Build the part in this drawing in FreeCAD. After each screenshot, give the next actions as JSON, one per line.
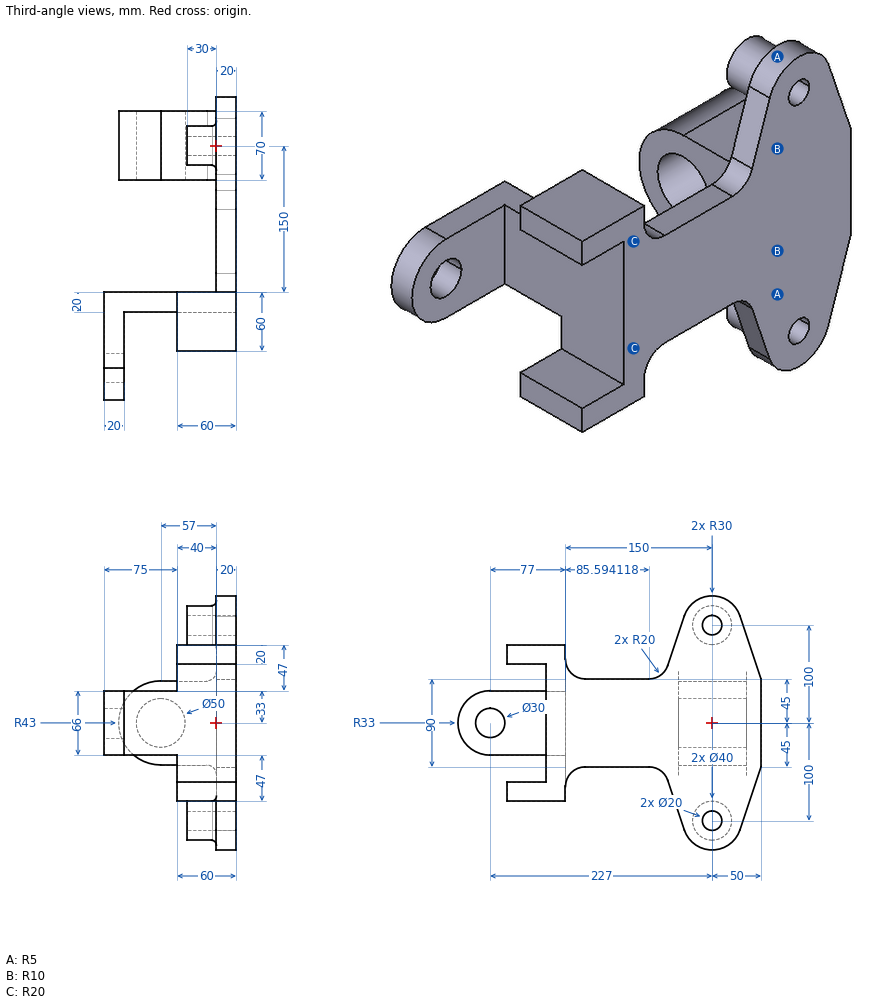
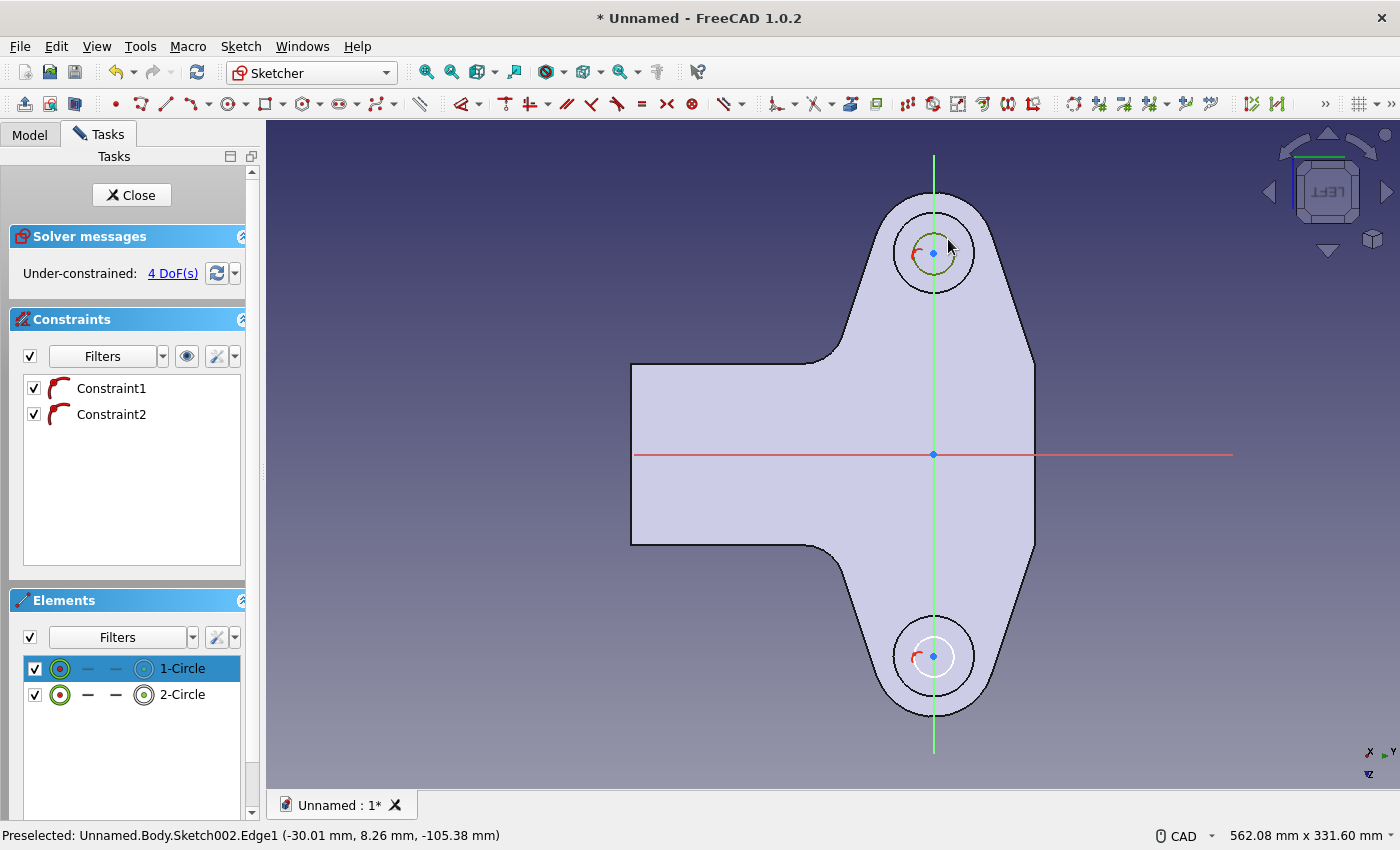
{"action": "left_click", "coordinate": [948, 643]}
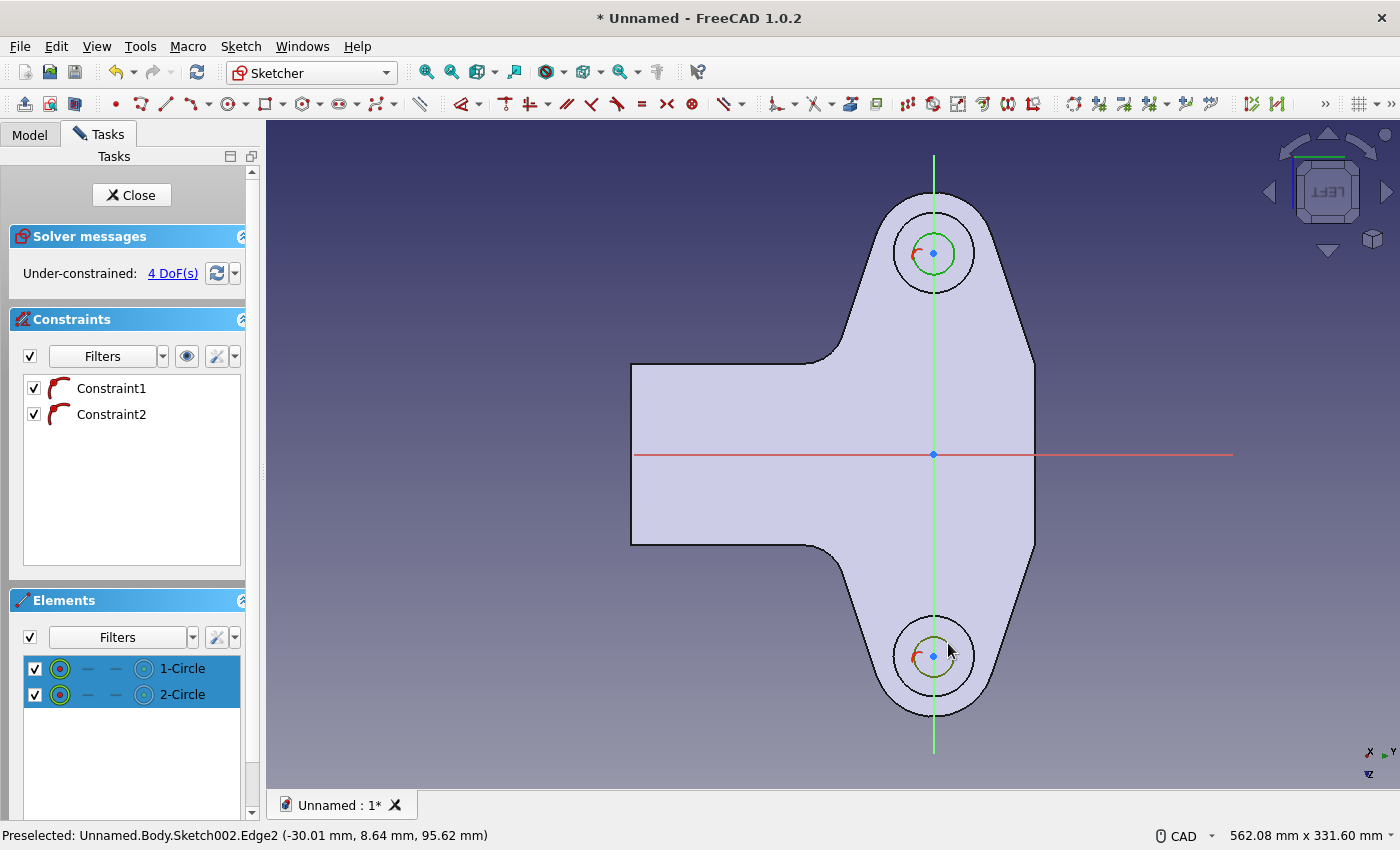
{"action": "key", "text": "e"}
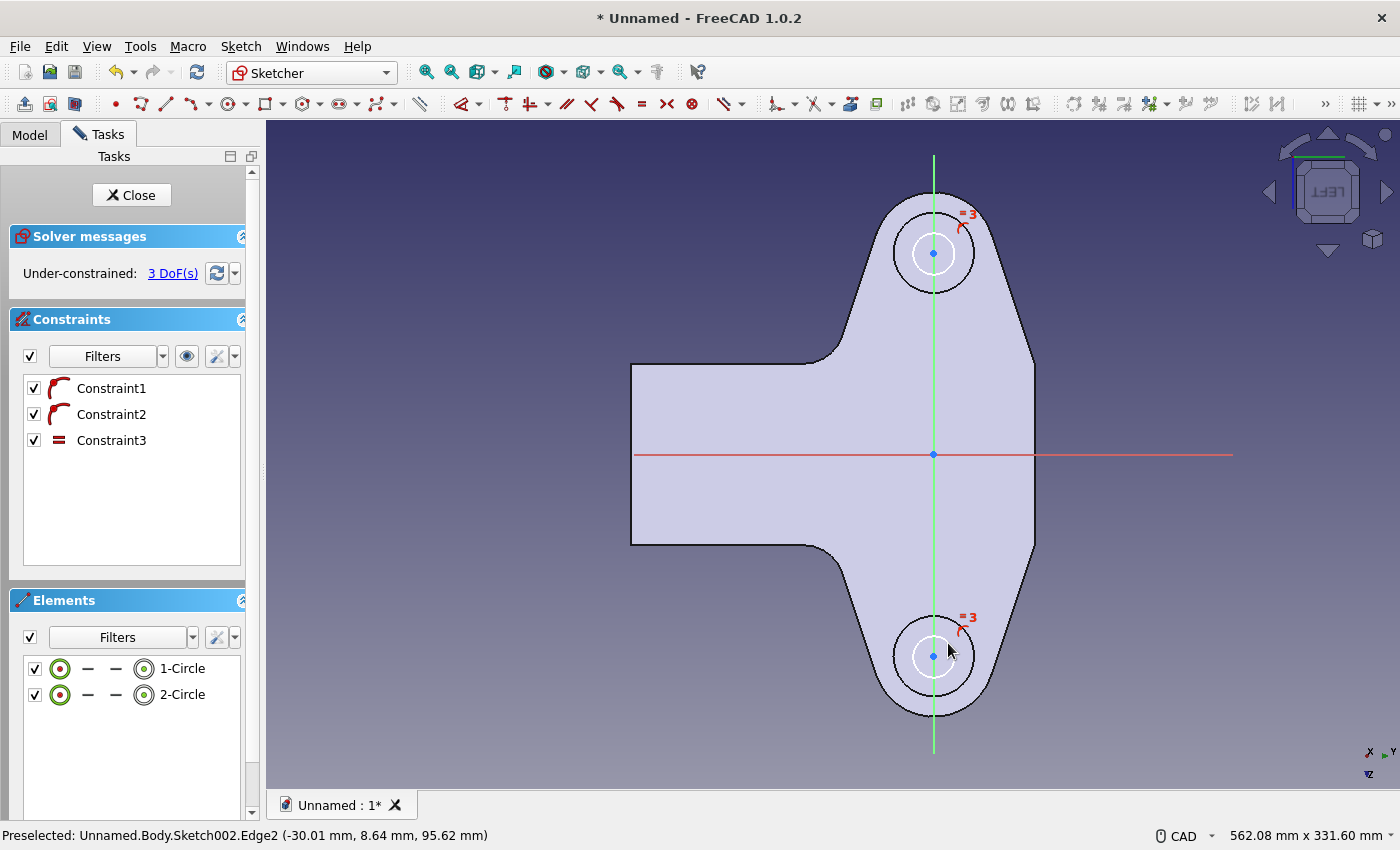
{"action": "key", "text": "d"}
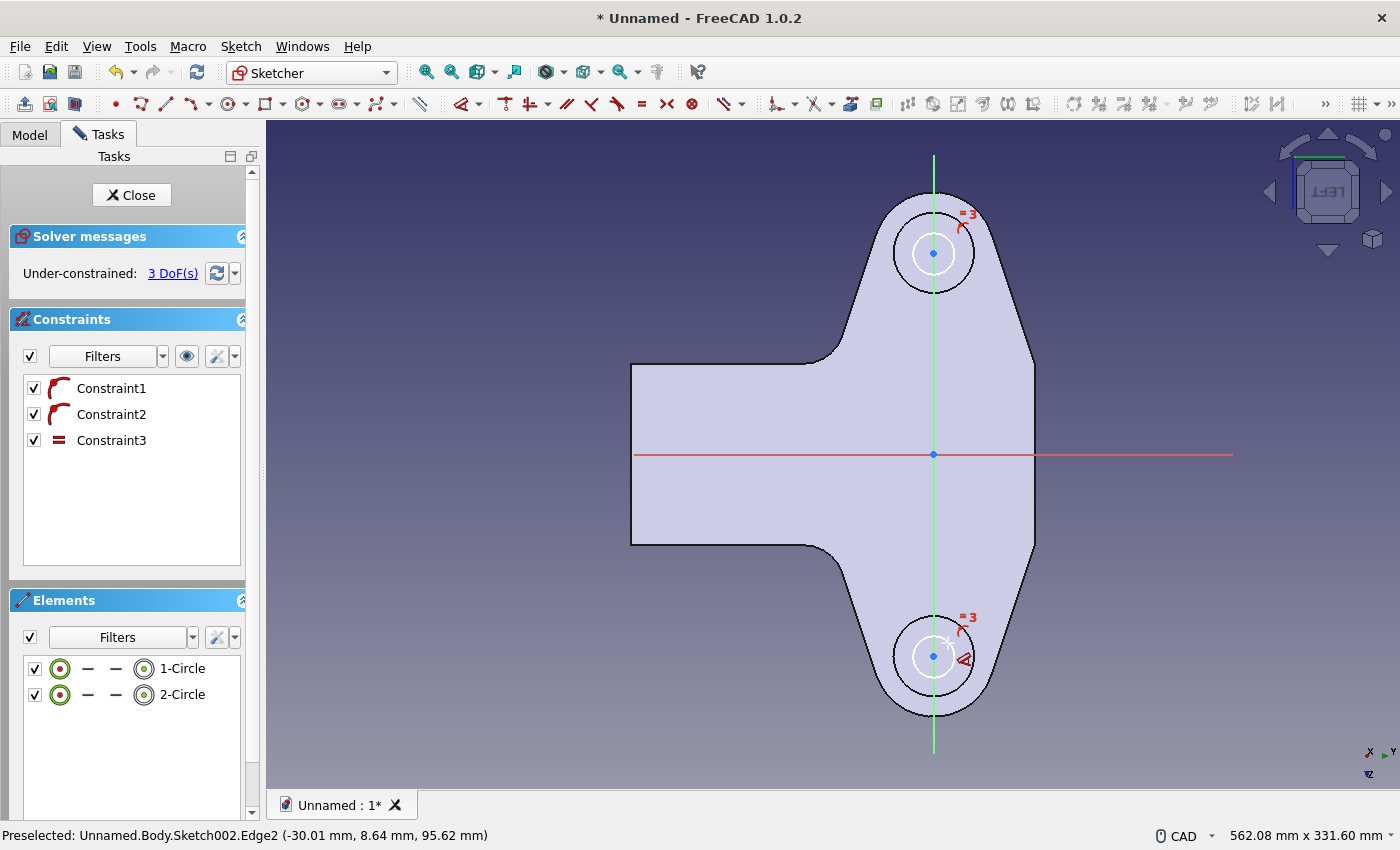
{"action": "left_click", "coordinate": [948, 239]}
{"action": "left_click", "coordinate": [970, 216]}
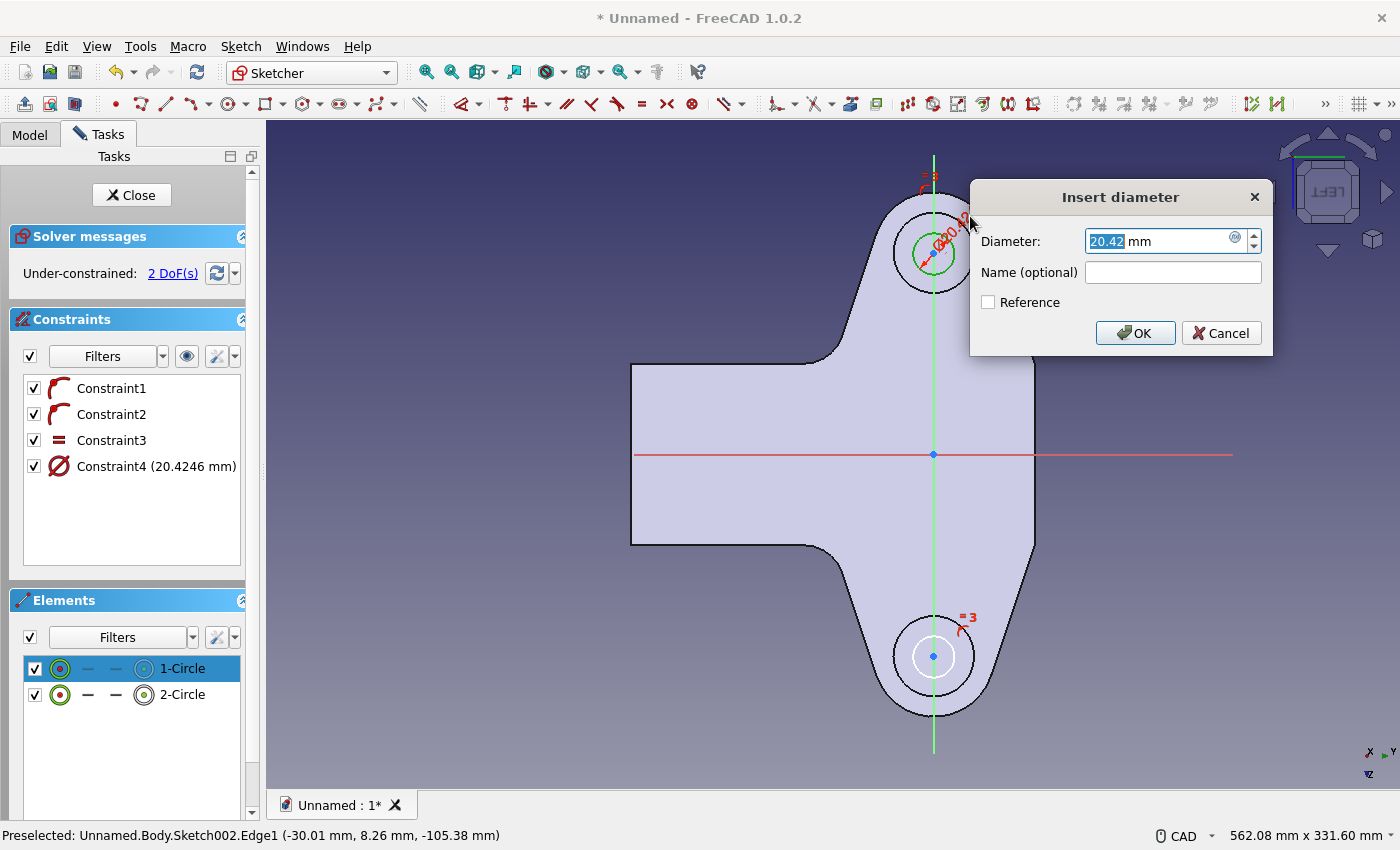
{"action": "type", "text": "20"}
{"action": "key", "text": "Return"}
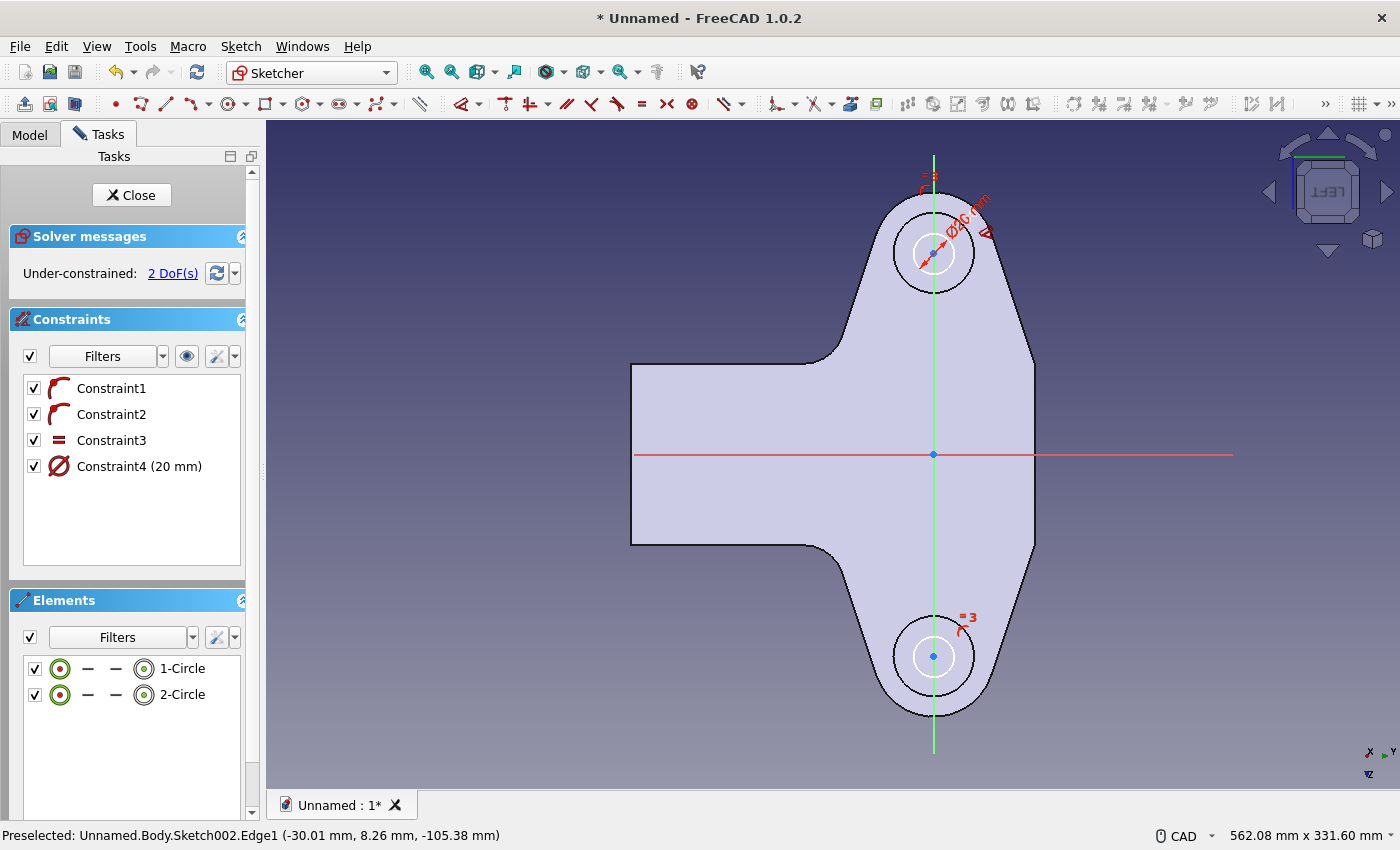
{"action": "left_click", "coordinate": [934, 254]}
{"action": "left_click", "coordinate": [968, 354]}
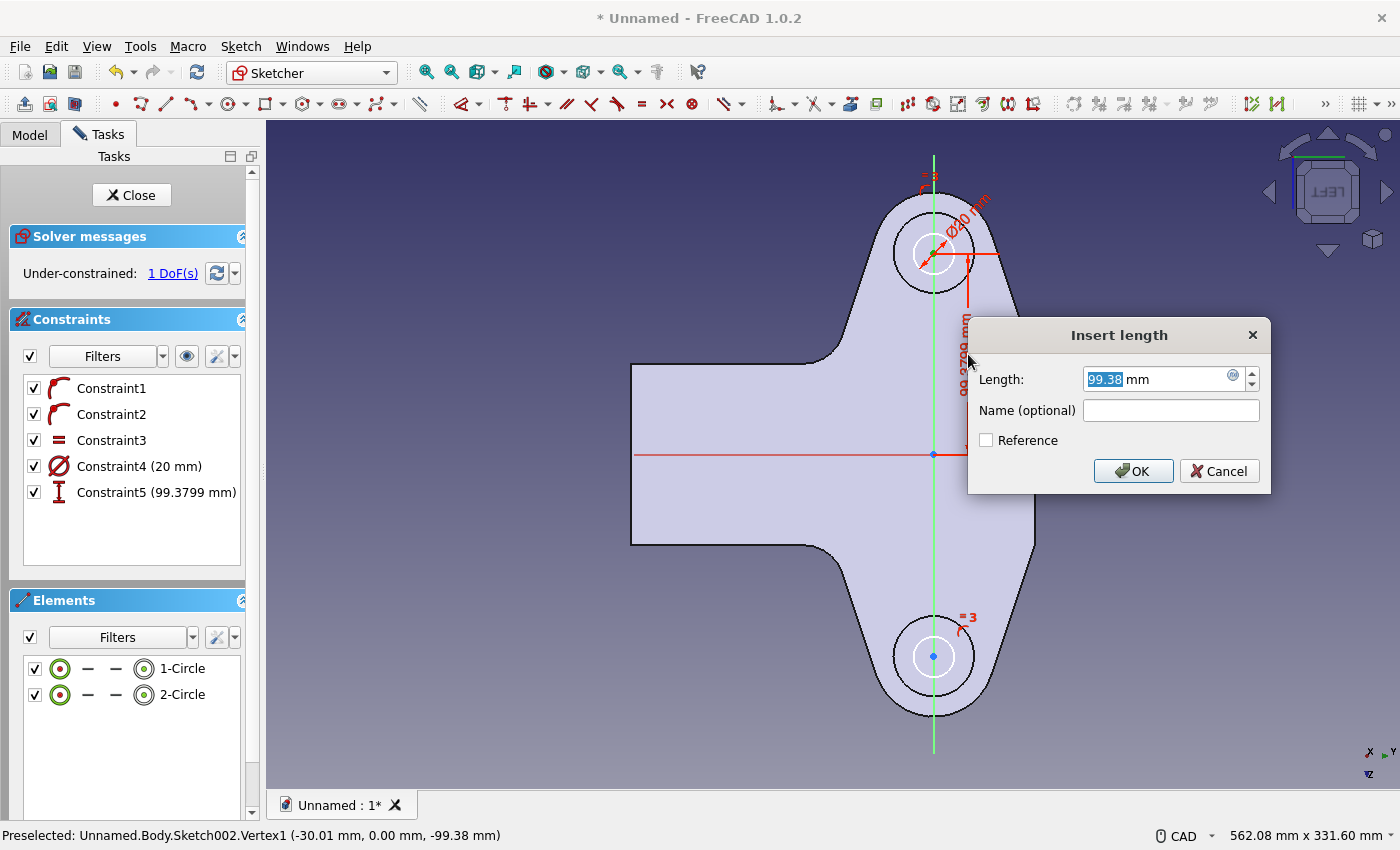
{"action": "type", "text": "100"}
{"action": "key", "text": "Return"}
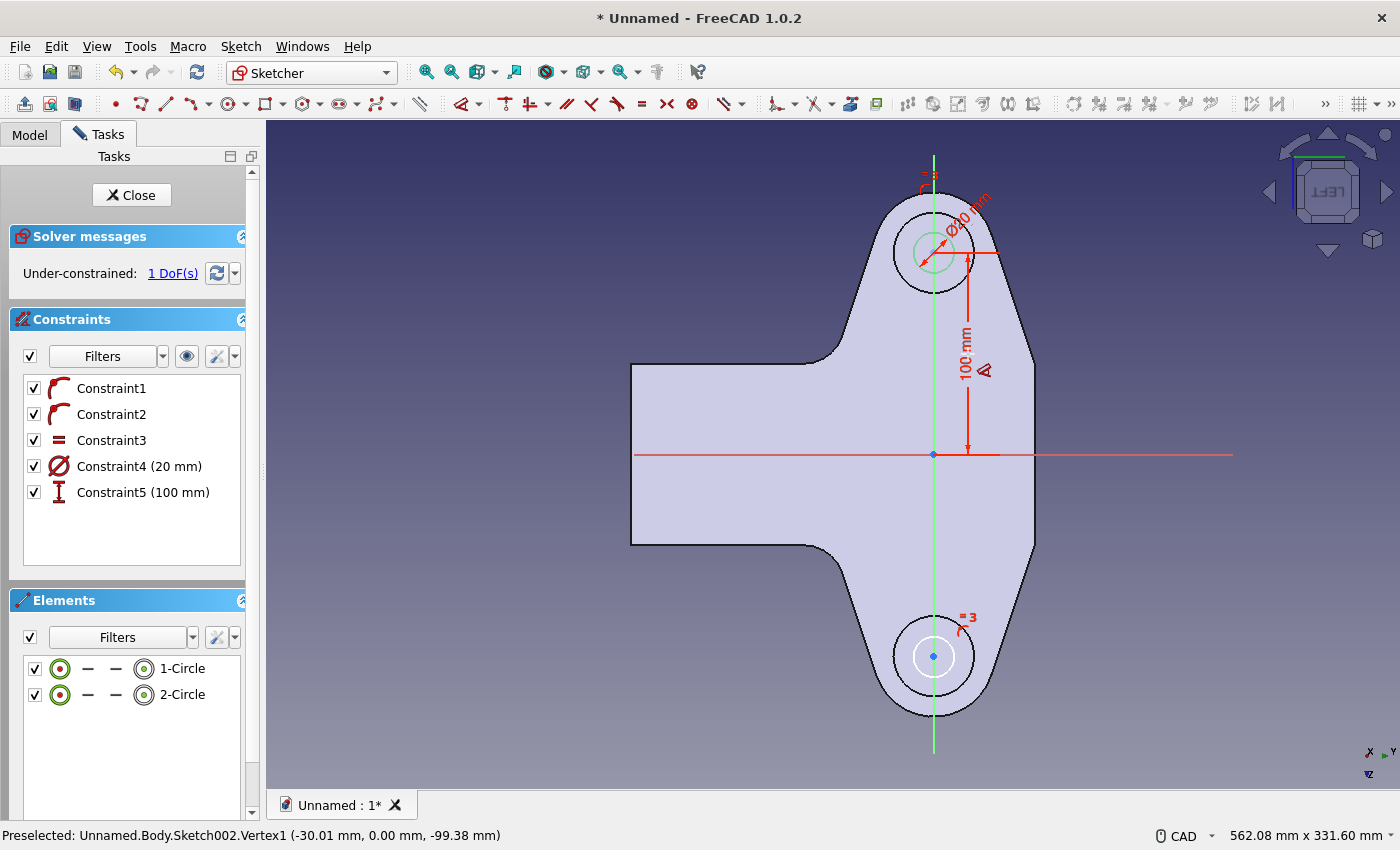
{"action": "left_click", "coordinate": [934, 657]}
{"action": "left_click", "coordinate": [968, 556]}